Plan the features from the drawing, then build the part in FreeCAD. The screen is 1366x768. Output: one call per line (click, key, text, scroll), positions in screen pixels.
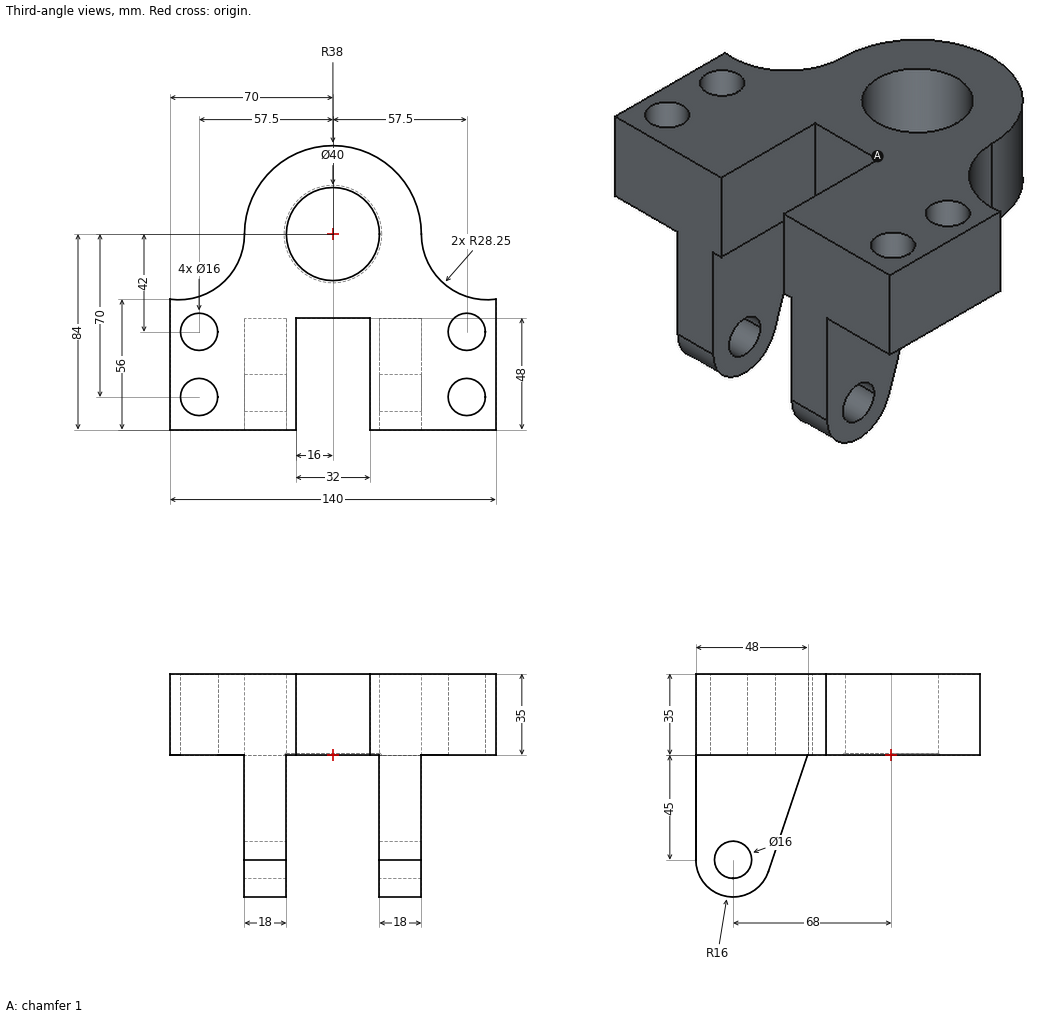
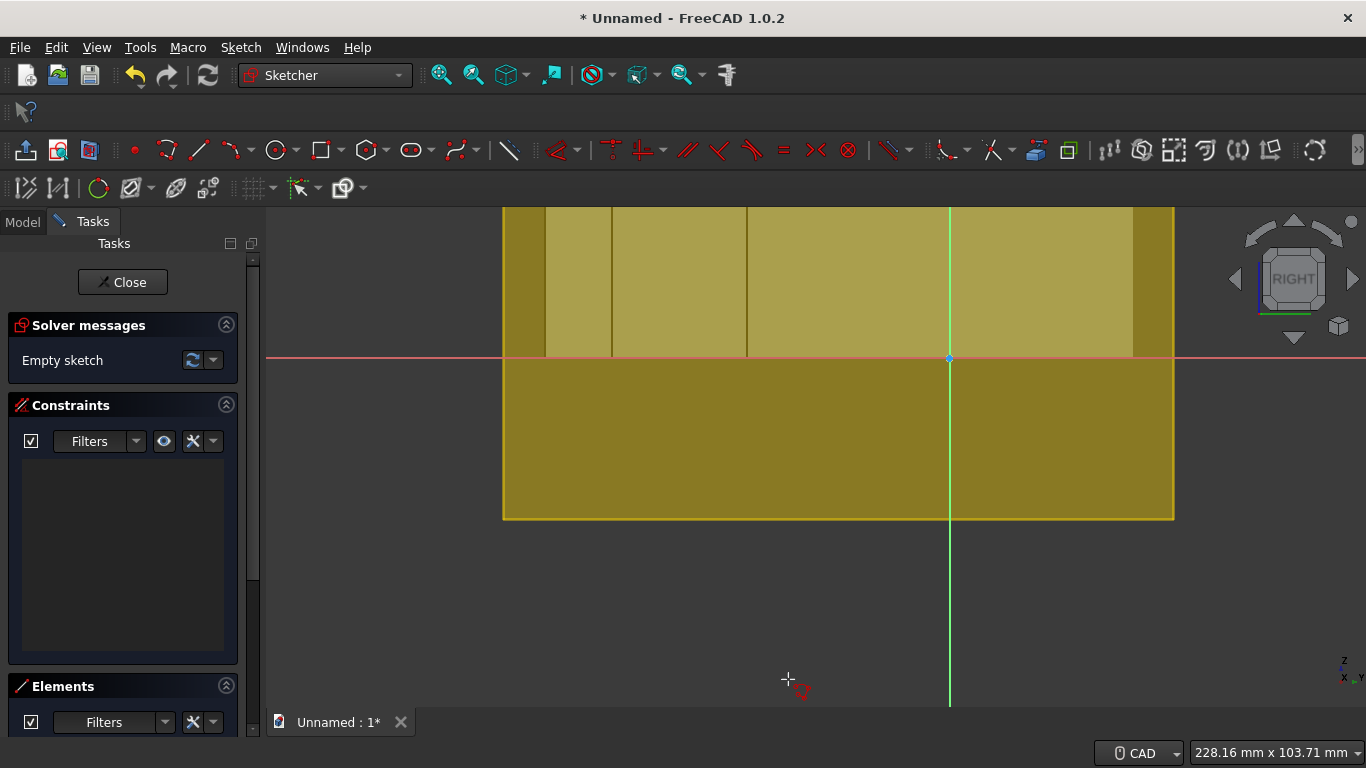
click(695, 600)
click(776, 358)
click(545, 367)
click(545, 575)
right_click(545, 575)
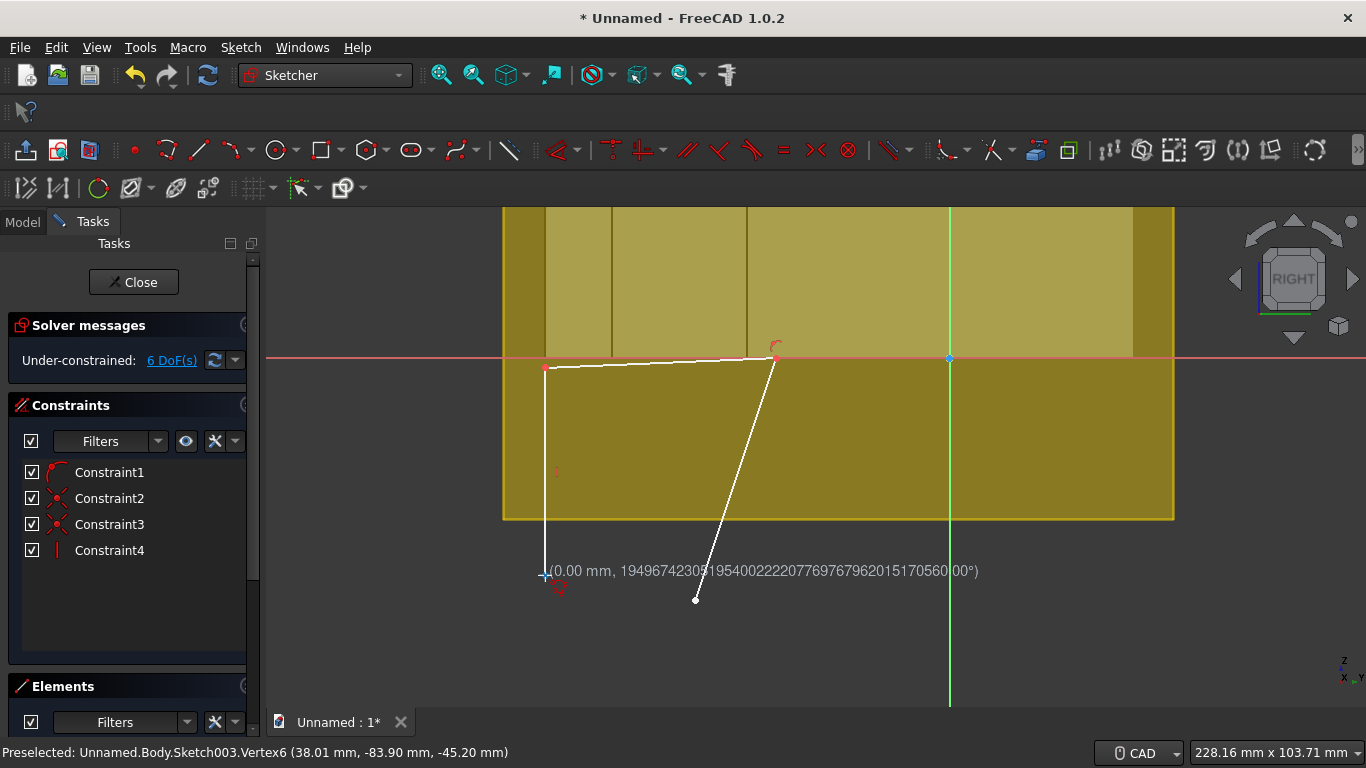
key(g)
key(3)
key(a)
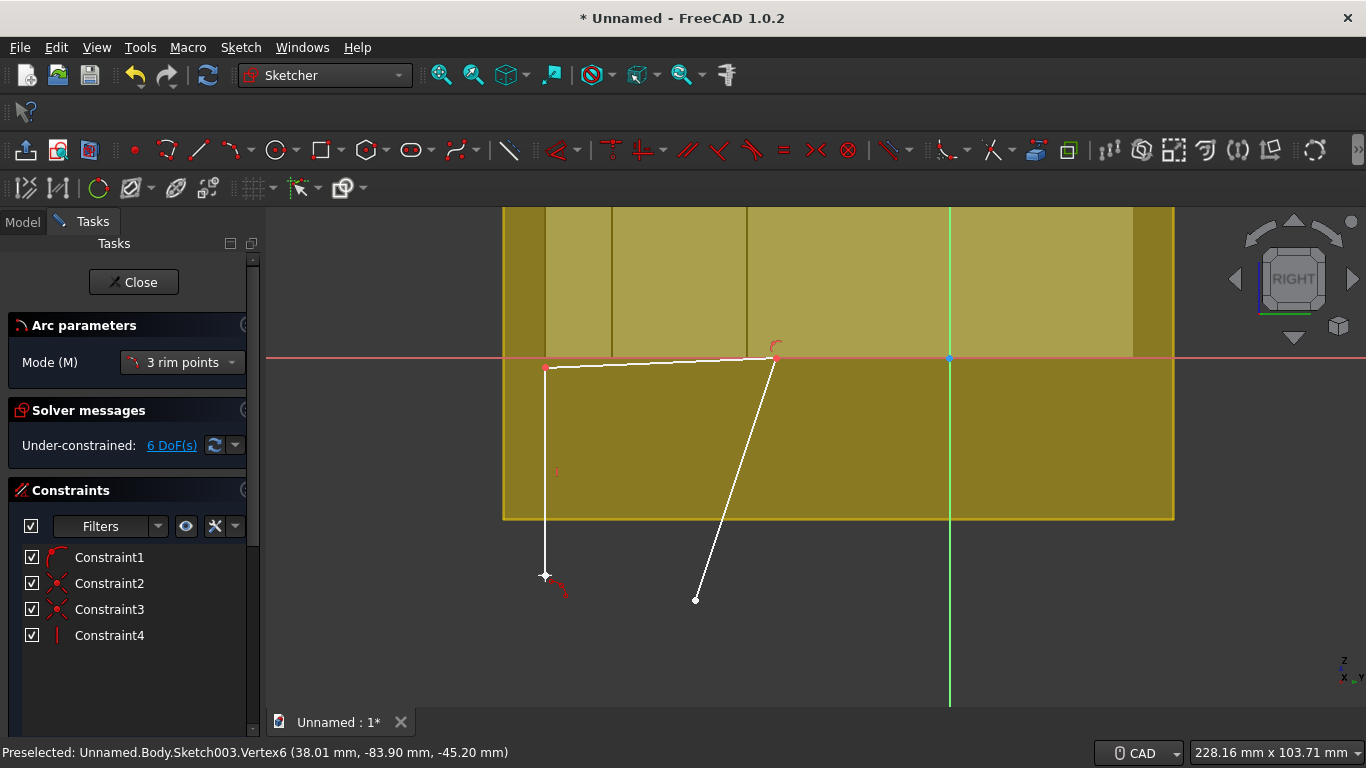
click(545, 576)
click(695, 601)
click(609, 651)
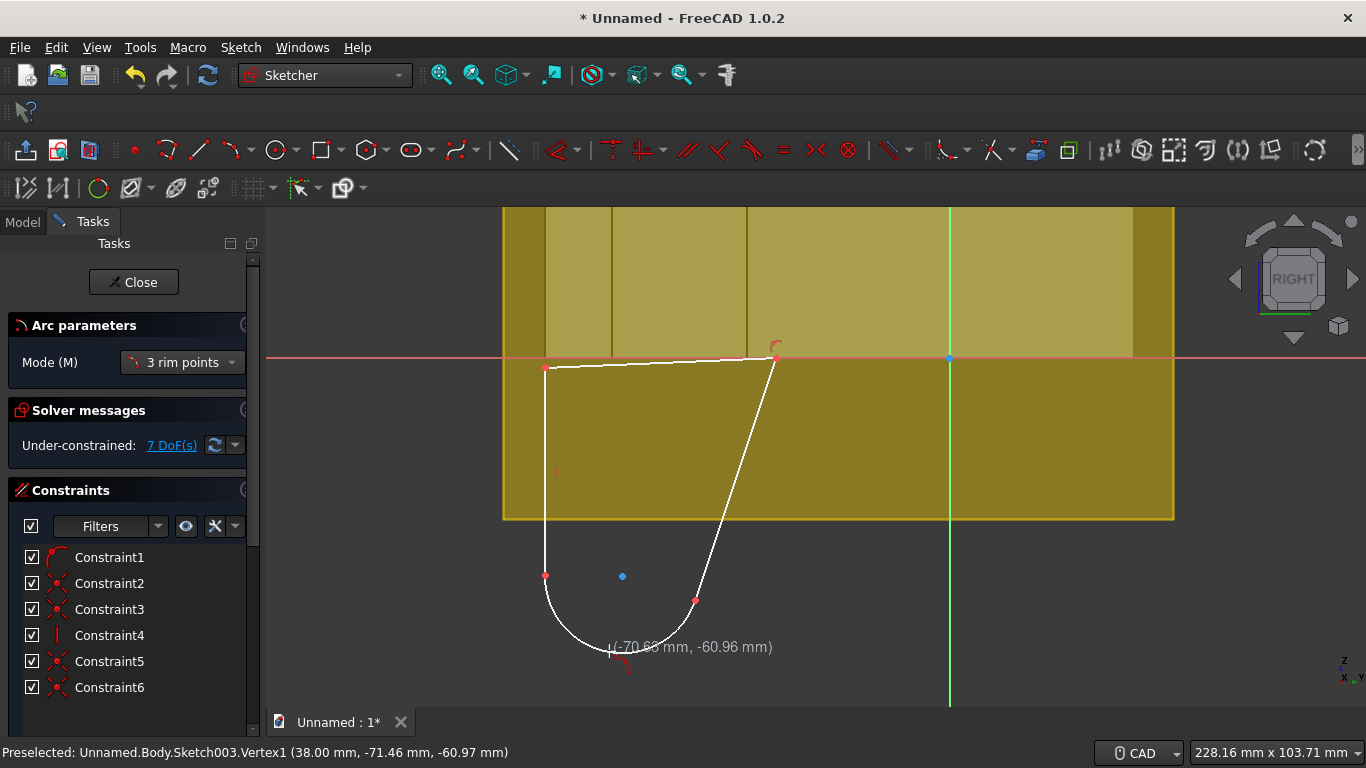
key(g)
key(c)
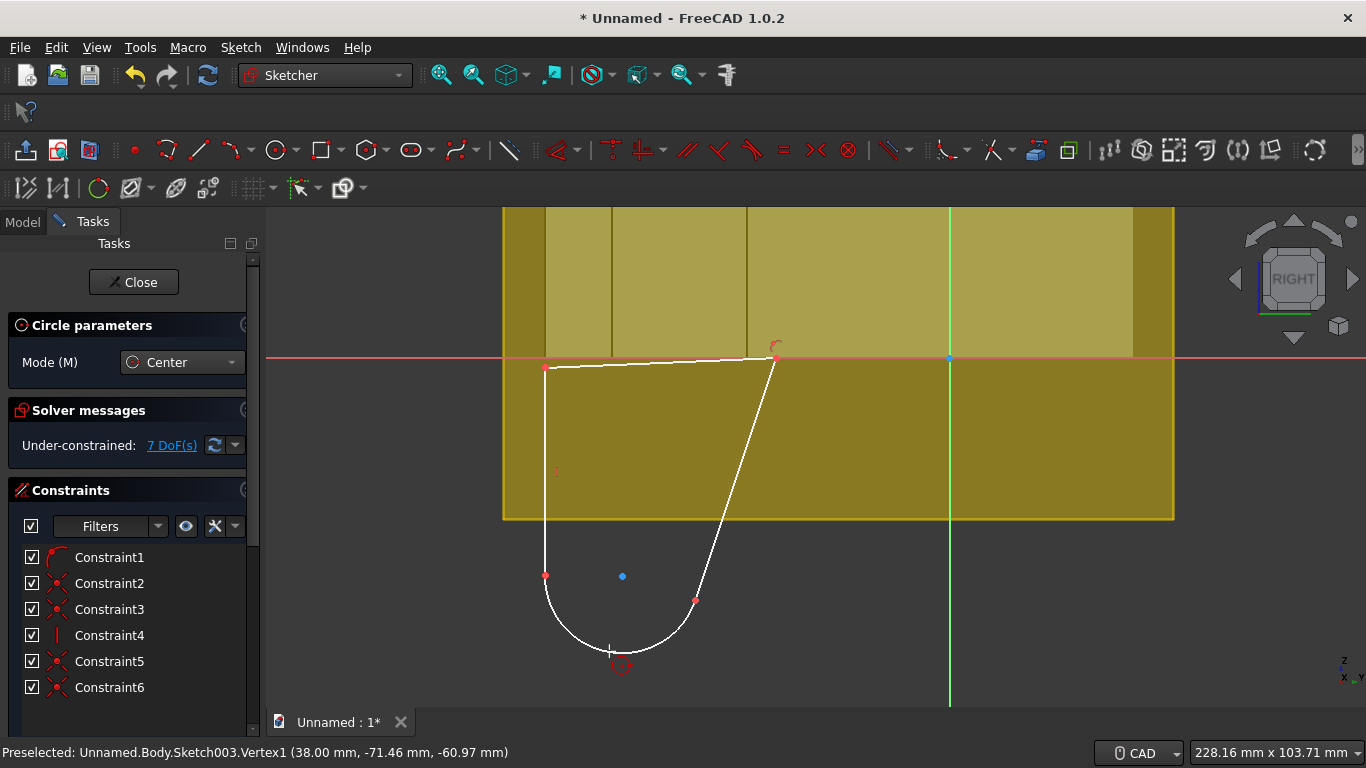
click(622, 575)
move(649, 548)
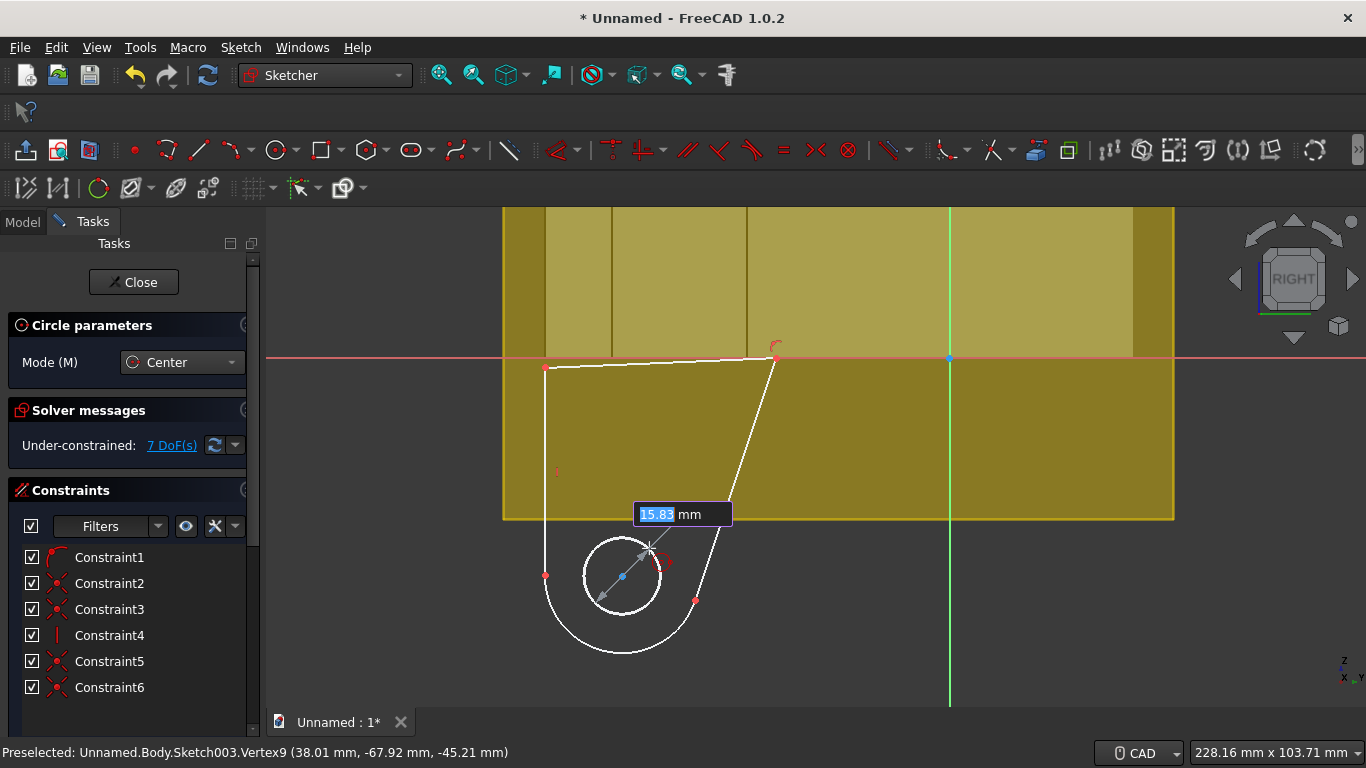
text(16)
key(Return)
key(Escape)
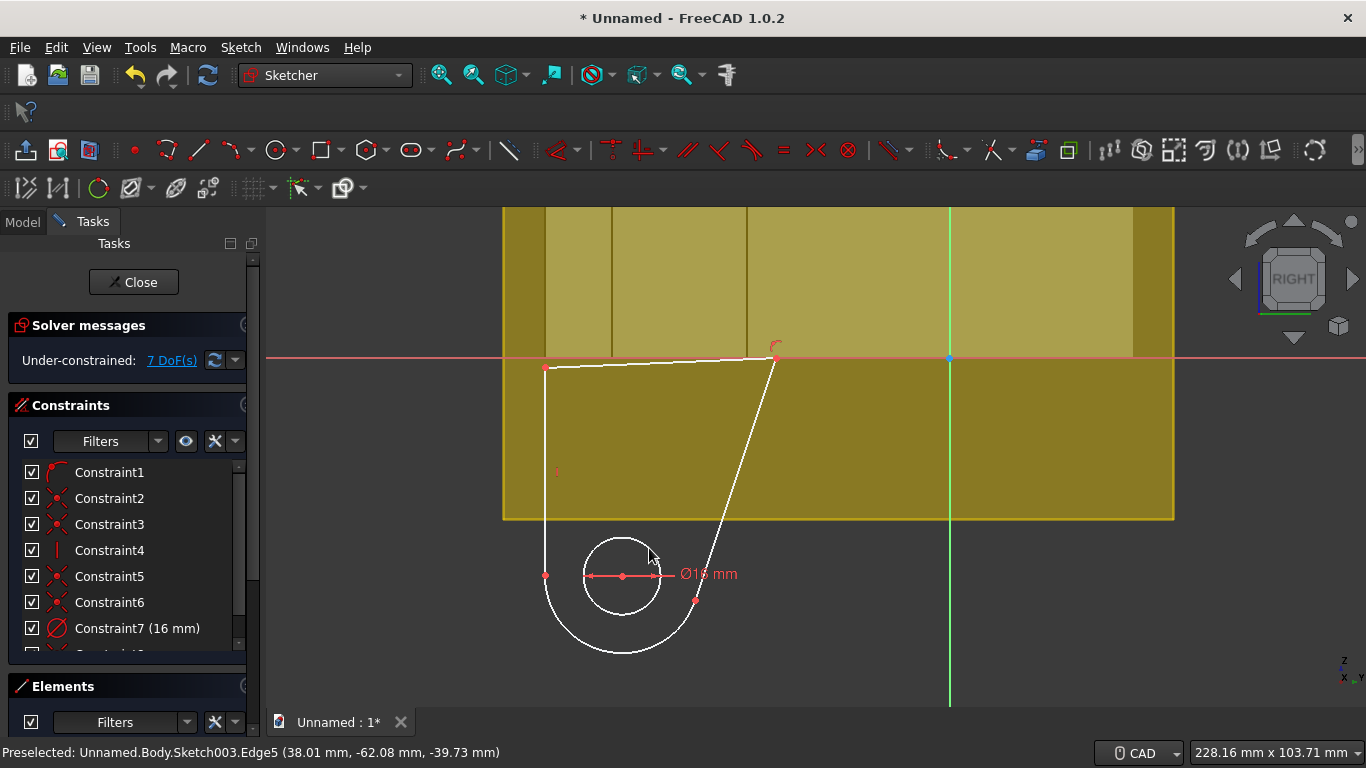
click(719, 528)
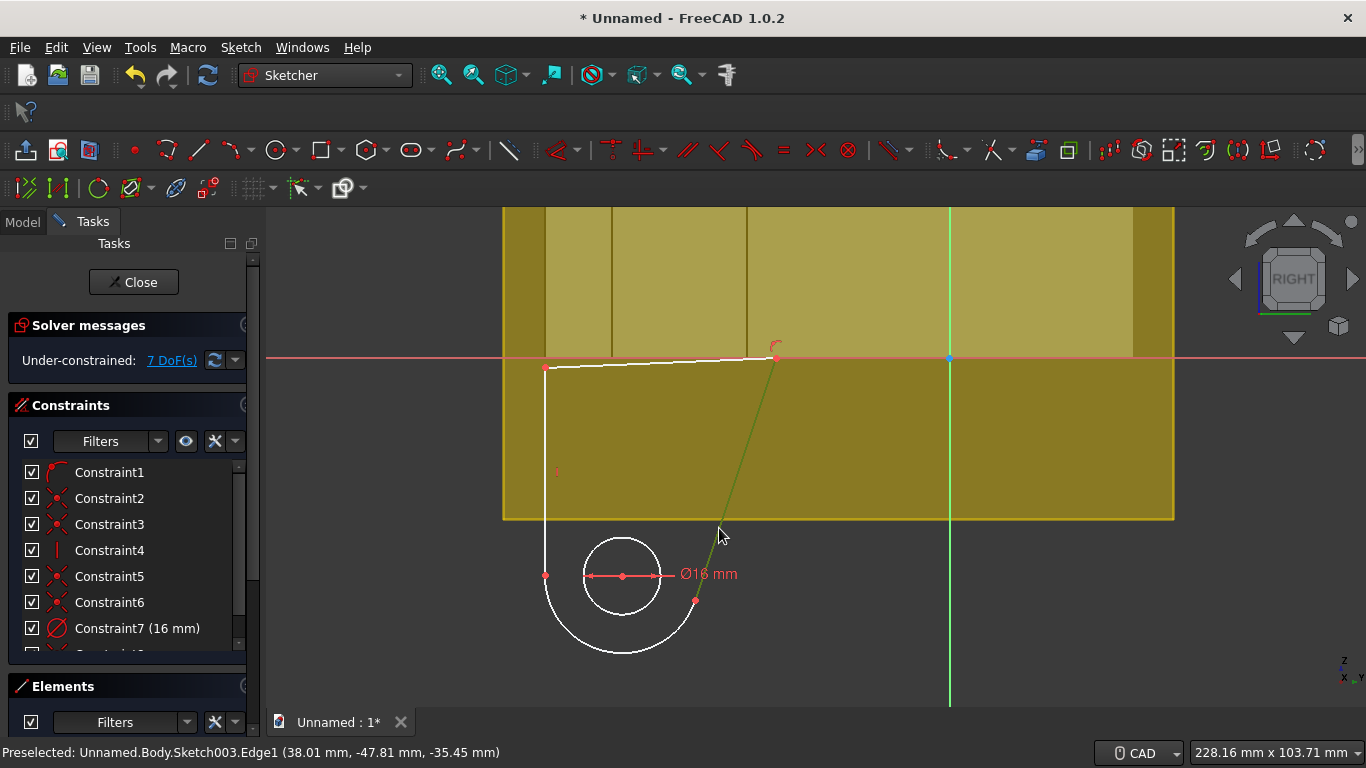
click(571, 634)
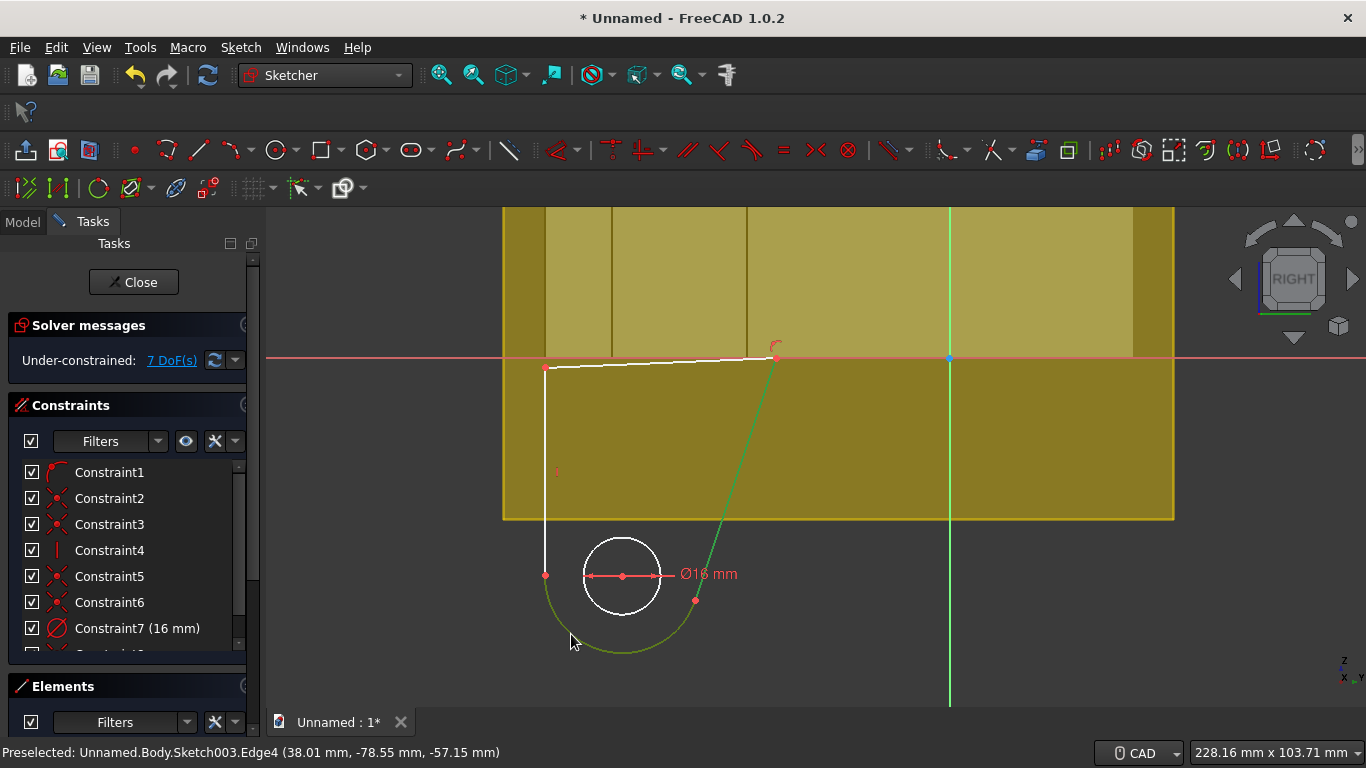
key(t)